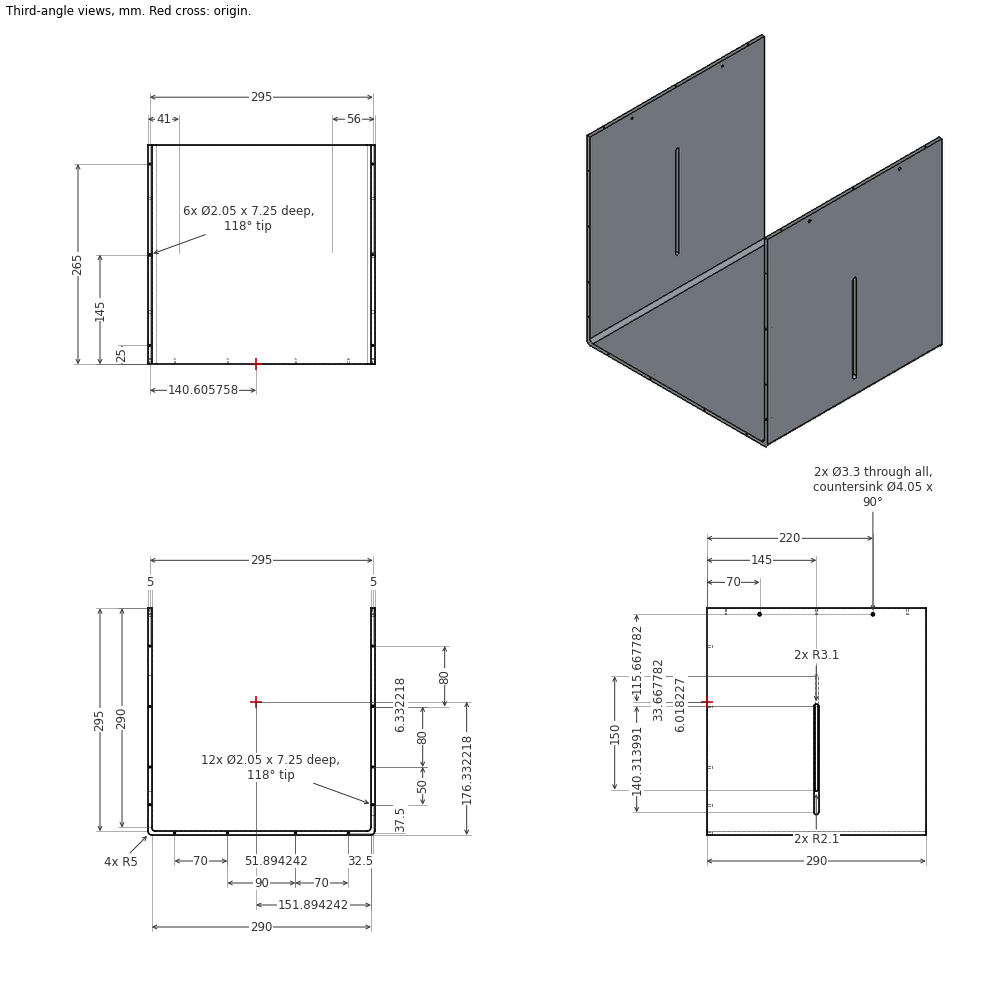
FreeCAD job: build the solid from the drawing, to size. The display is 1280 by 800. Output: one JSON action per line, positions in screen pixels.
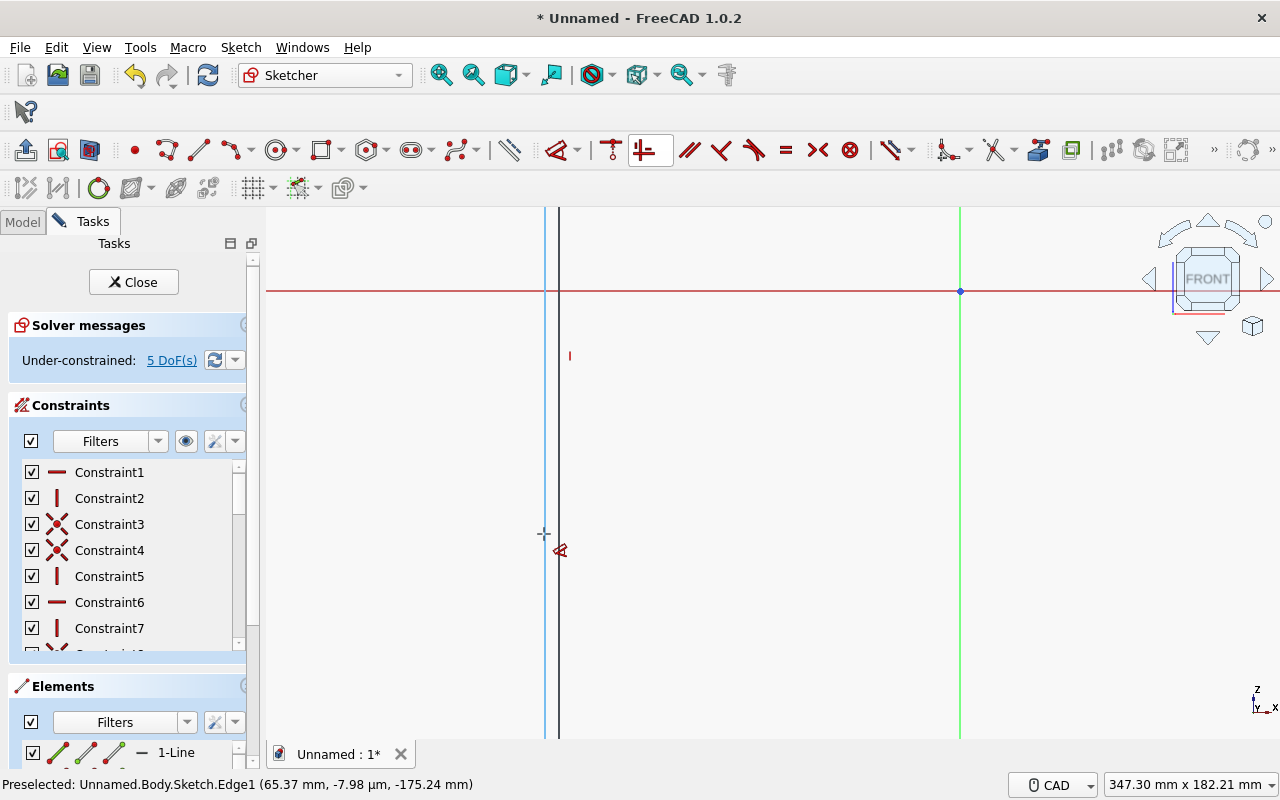
{"action": "left_click", "coordinate": [545, 532]}
{"action": "left_click", "coordinate": [511, 473]}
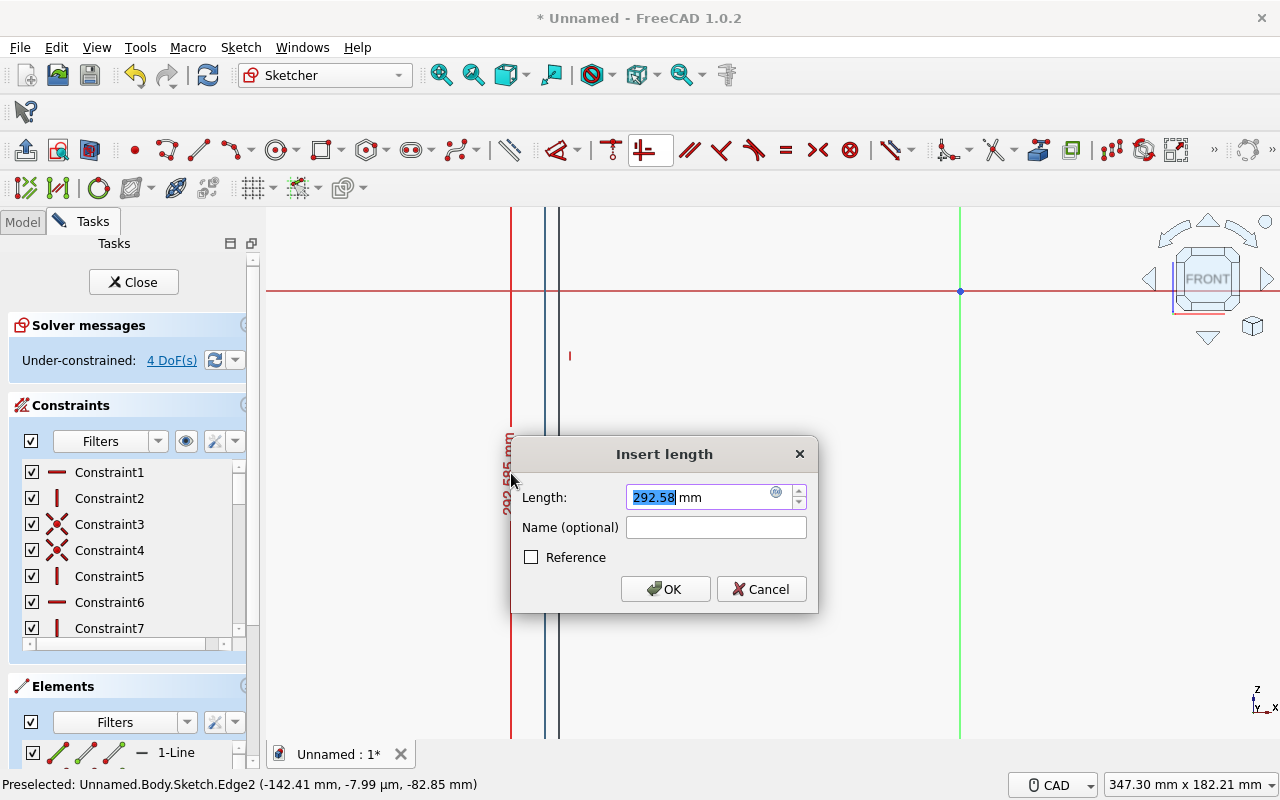
{"action": "type", "text": "295"}
{"action": "key", "text": "Return"}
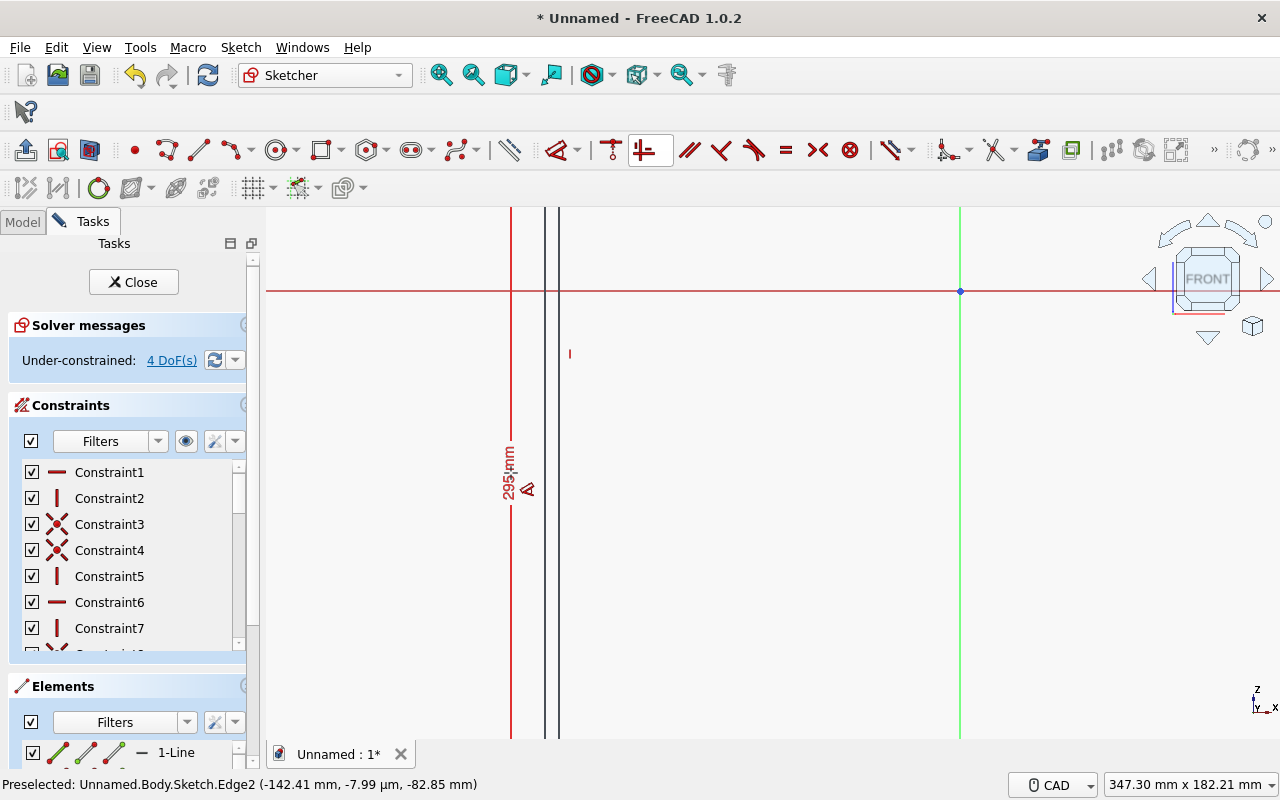
{"action": "left_click", "coordinate": [559, 526]}
{"action": "left_click", "coordinate": [525, 364]}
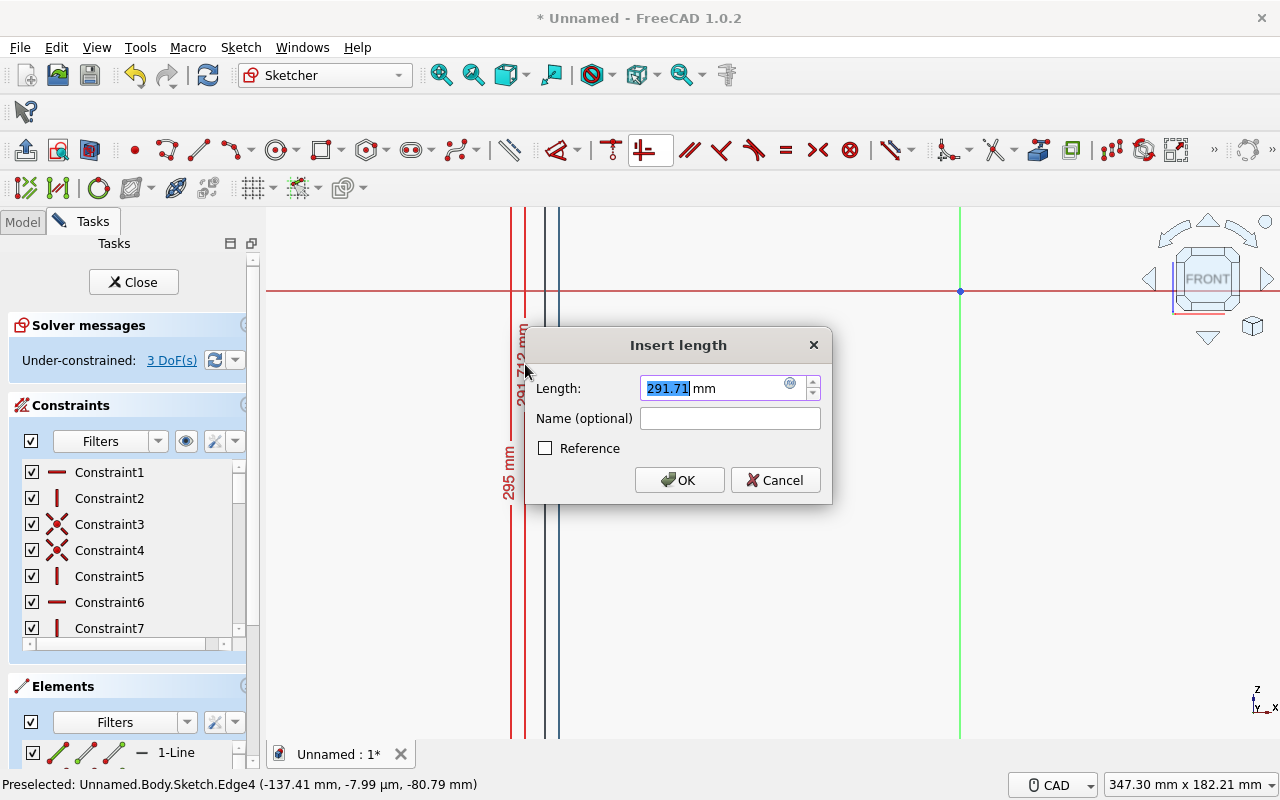
{"action": "type", "text": "290"}
{"action": "key", "text": "Return"}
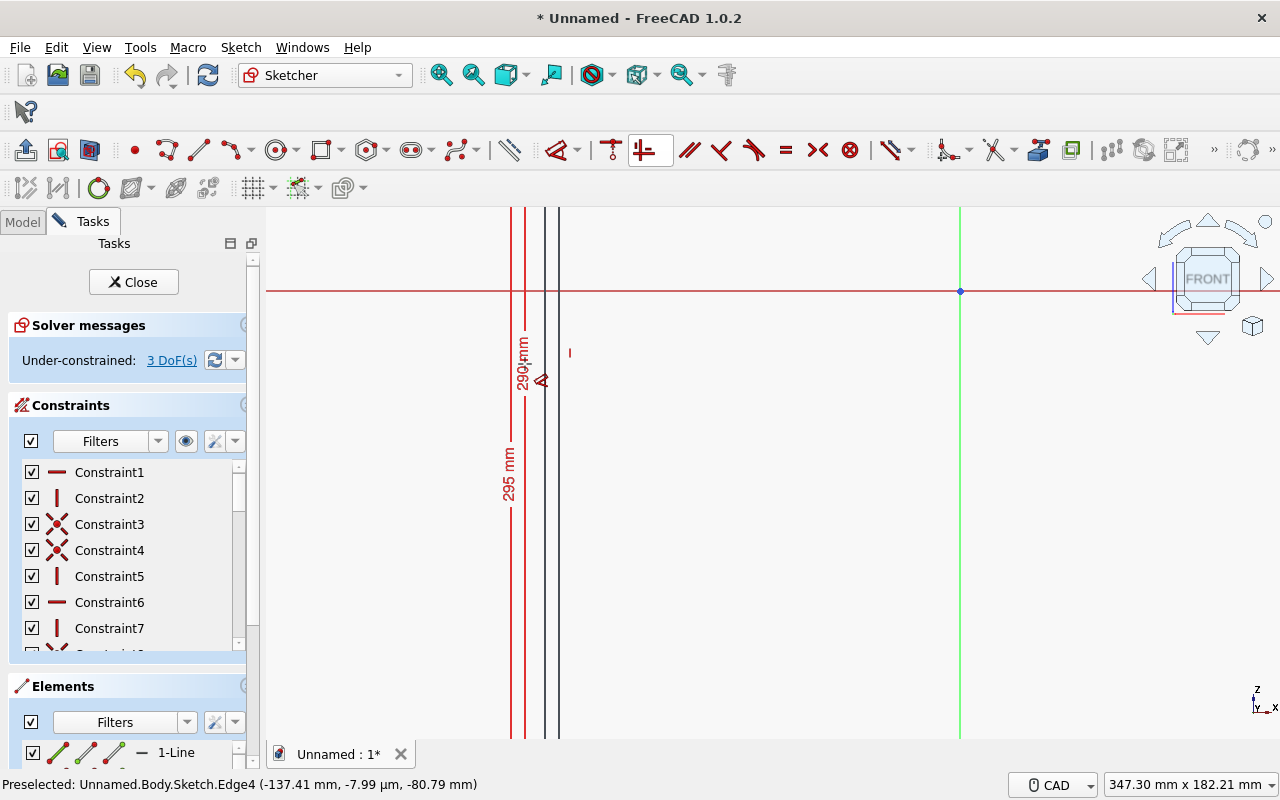
{"action": "scroll", "coordinate": [544, 534], "scroll_direction": "down", "scroll_amount": 5}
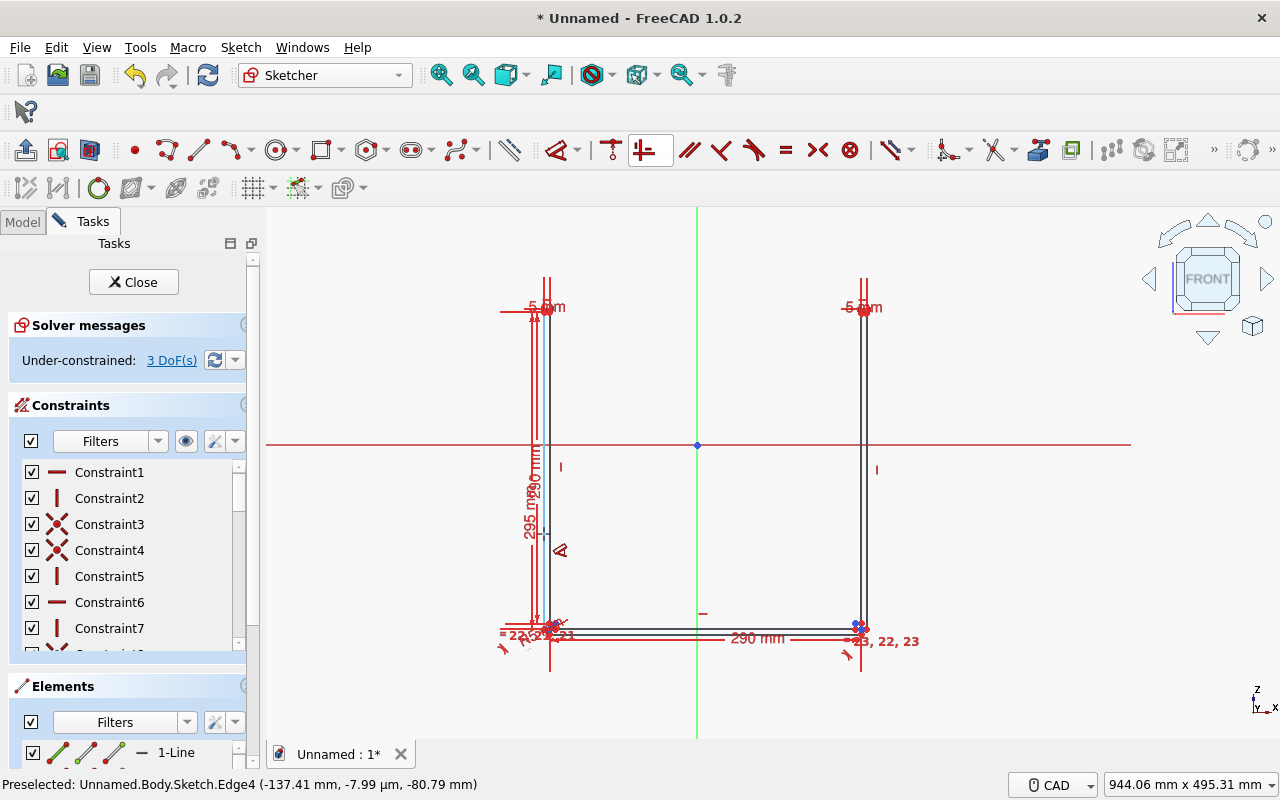
{"action": "scroll", "coordinate": [861, 531], "scroll_direction": "up", "scroll_amount": 5}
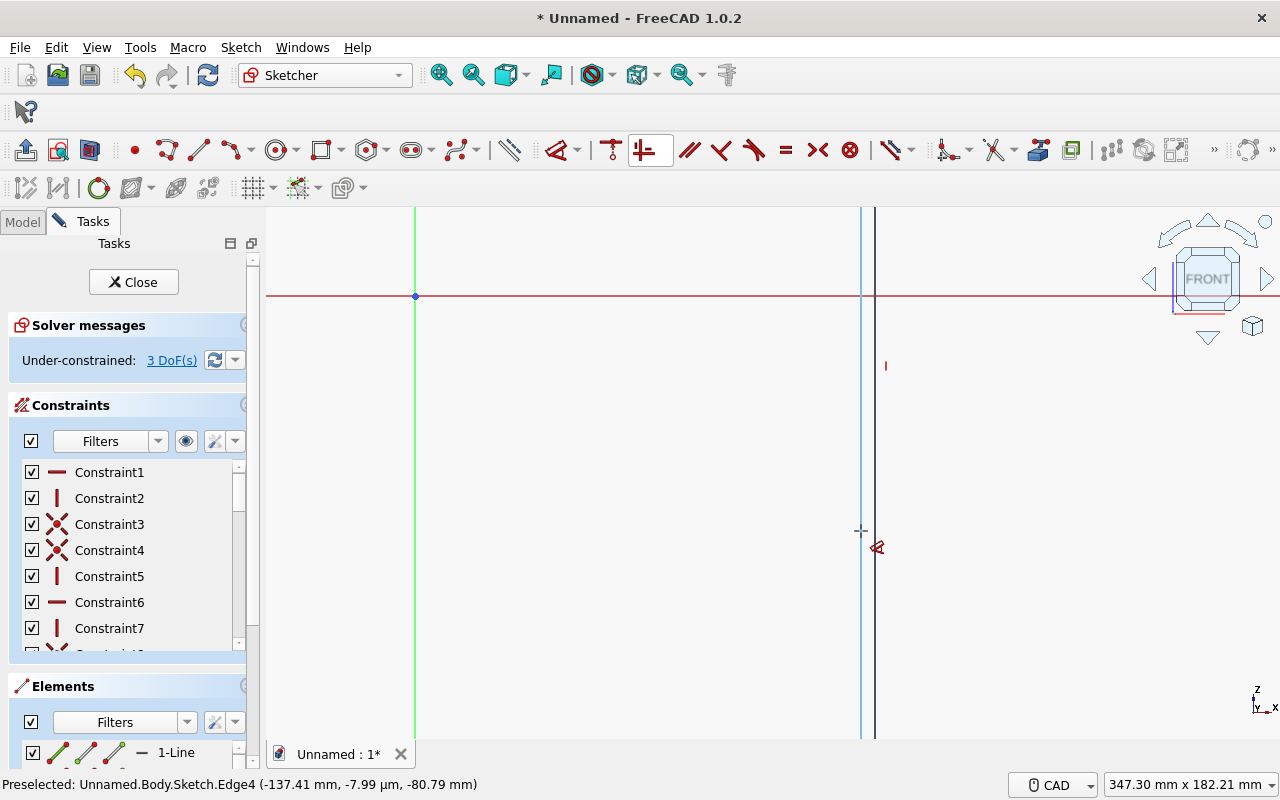
{"action": "left_click", "coordinate": [861, 529]}
{"action": "left_click", "coordinate": [895, 473]}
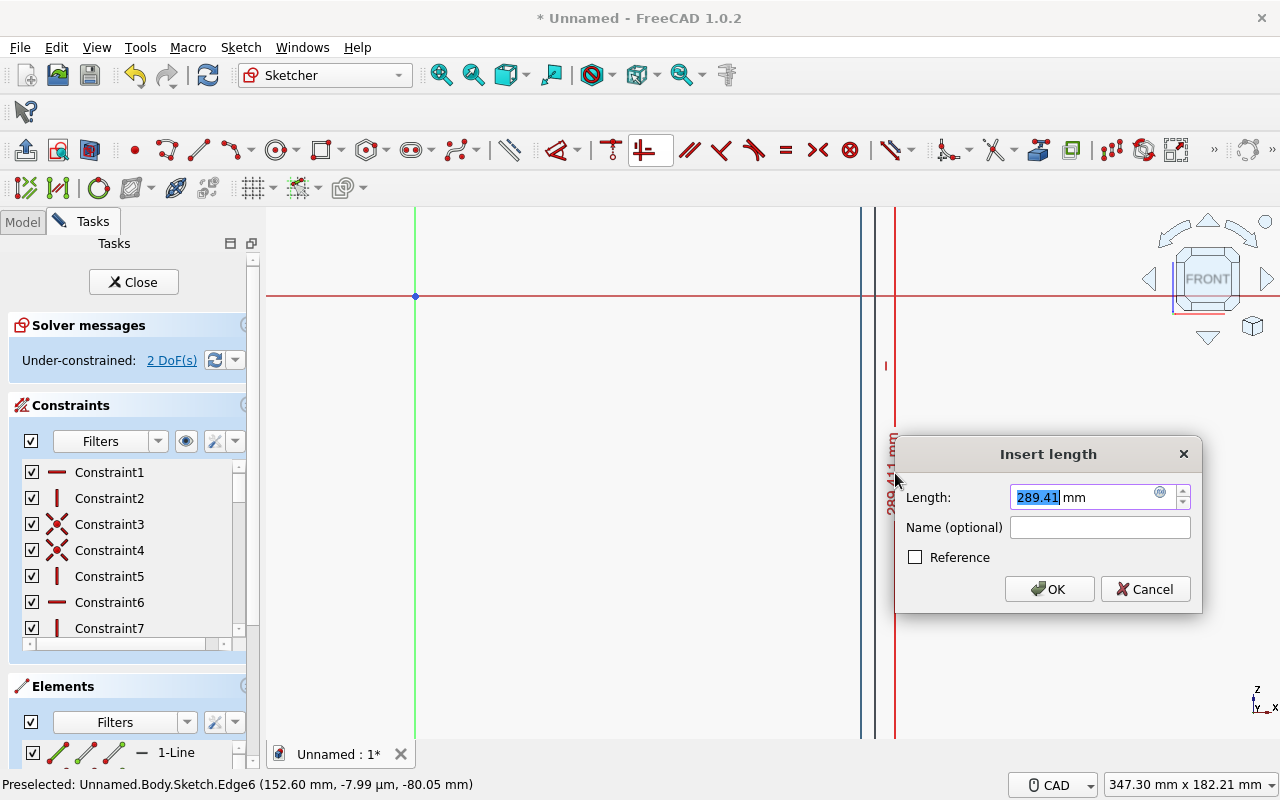
{"action": "type", "text": "290"}
{"action": "key", "text": "Return"}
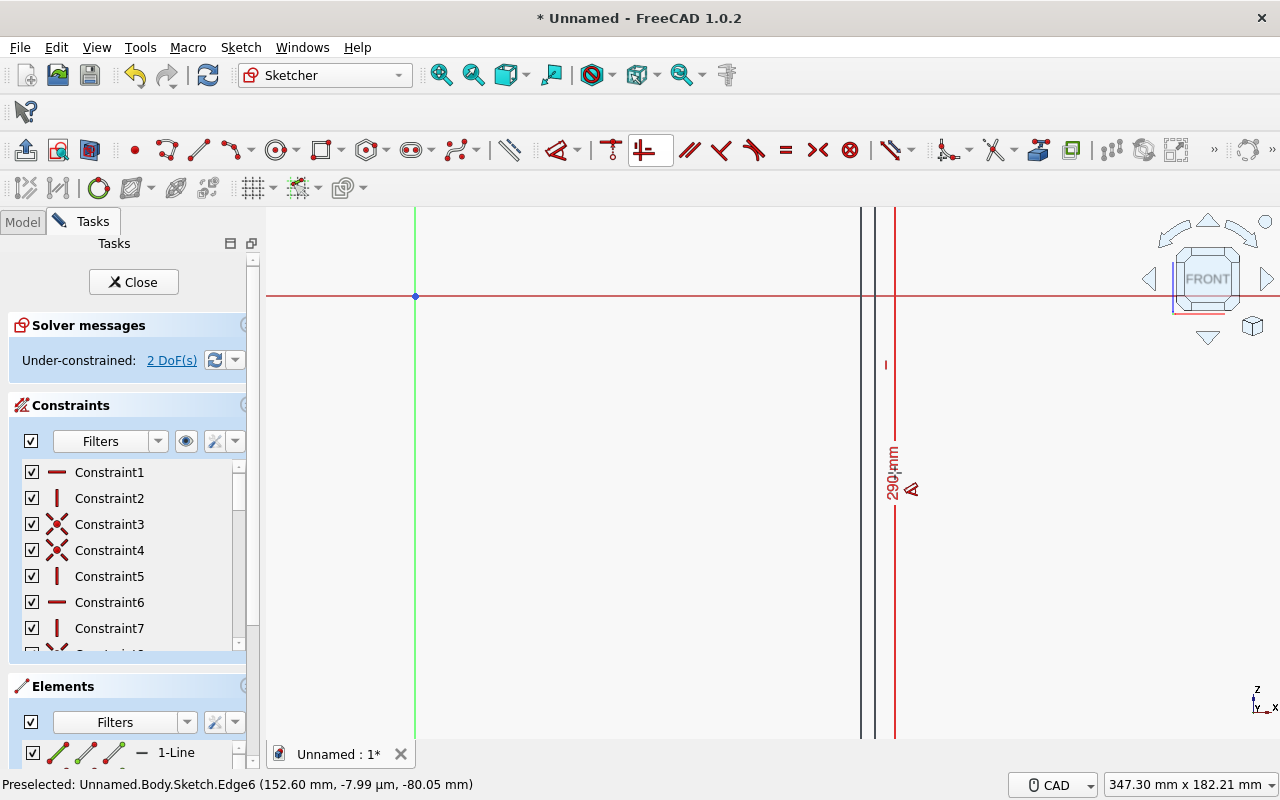
{"action": "scroll", "coordinate": [861, 531], "scroll_direction": "down", "scroll_amount": 5}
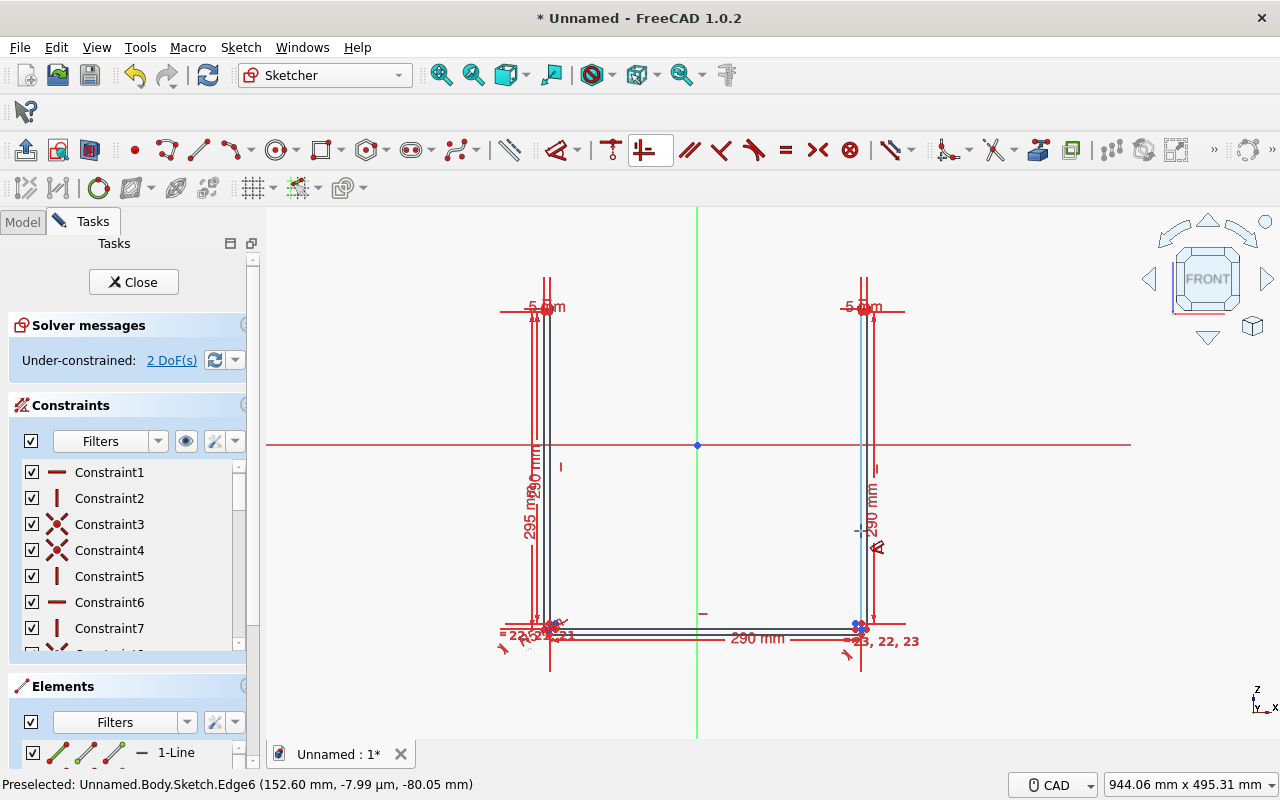
{"action": "scroll", "coordinate": [861, 635], "scroll_direction": "up", "scroll_amount": 5}